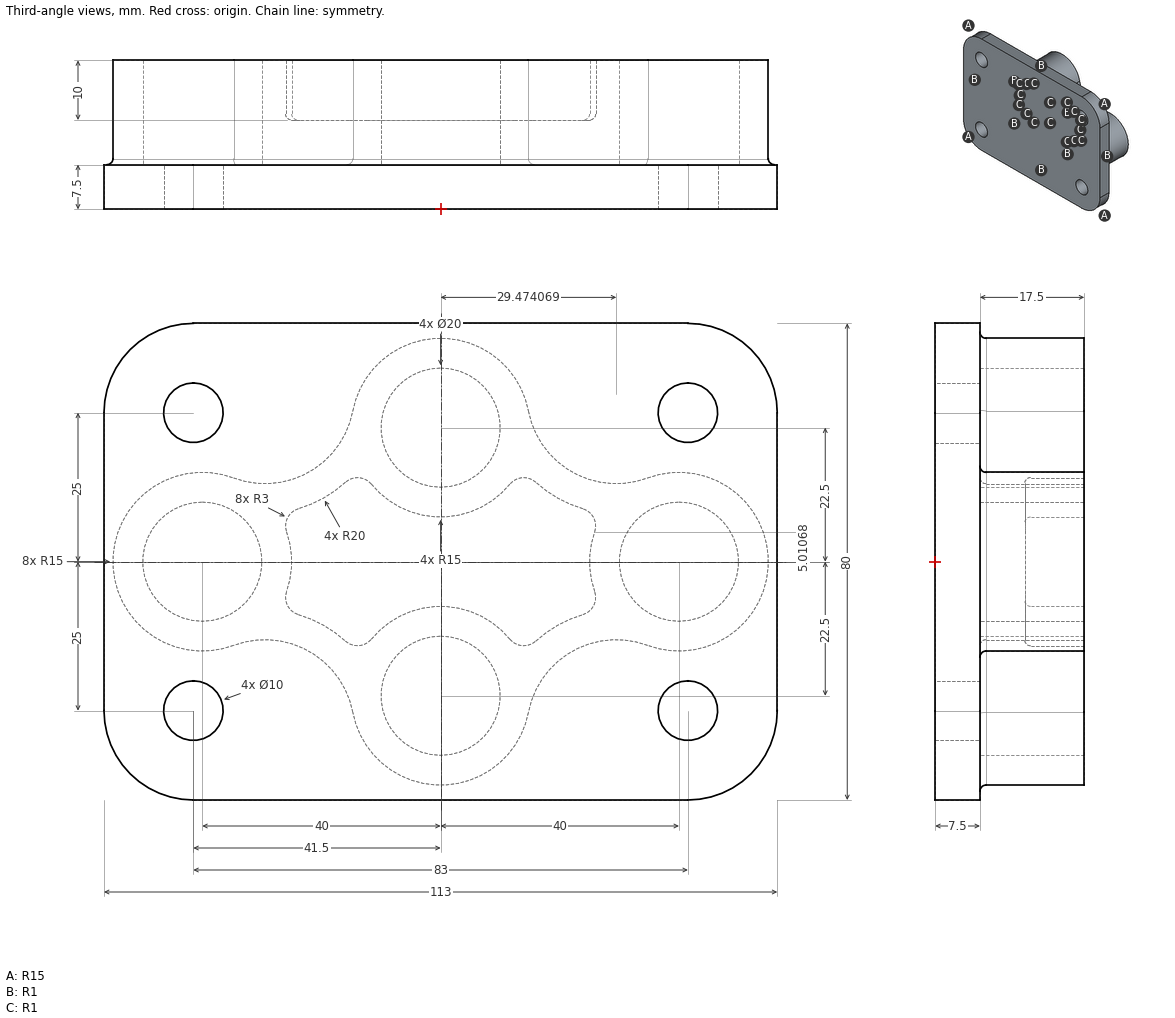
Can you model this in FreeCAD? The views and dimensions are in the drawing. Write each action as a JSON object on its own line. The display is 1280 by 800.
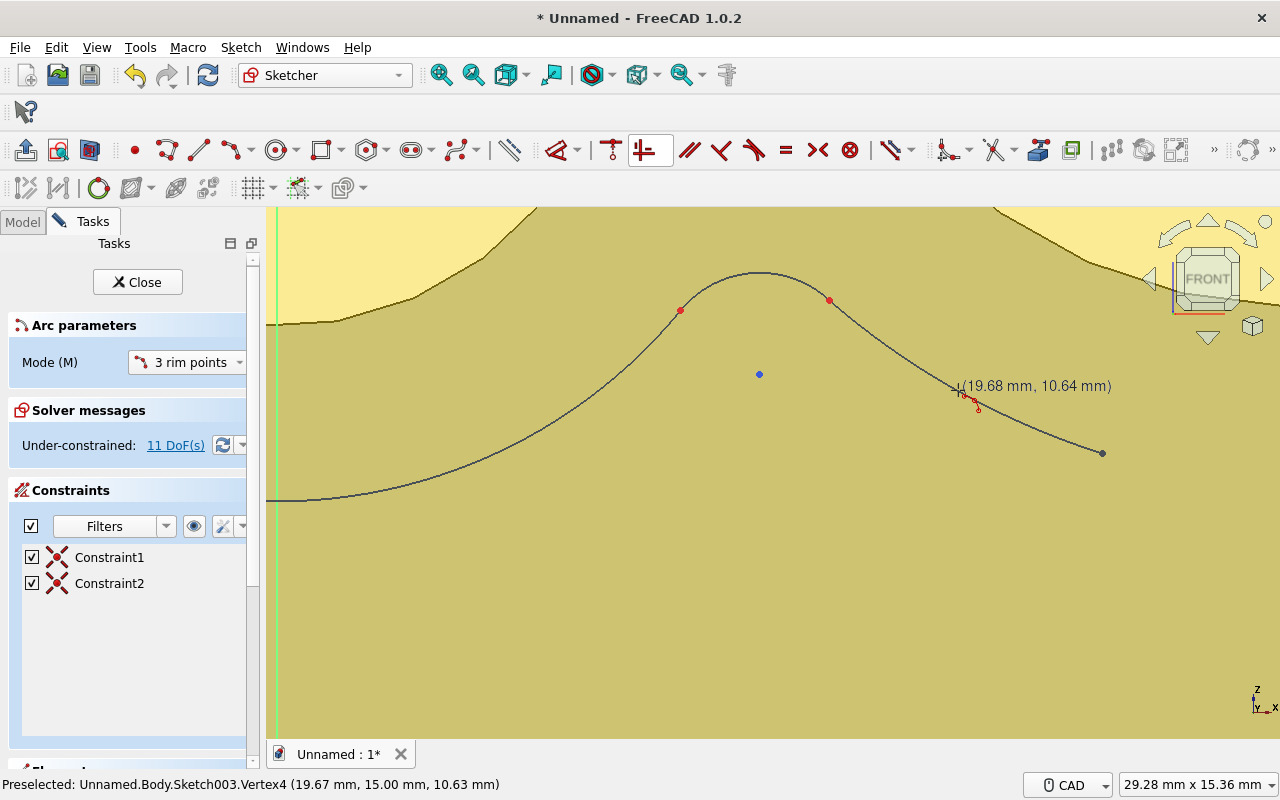
{"action": "left_click", "coordinate": [1102, 453]}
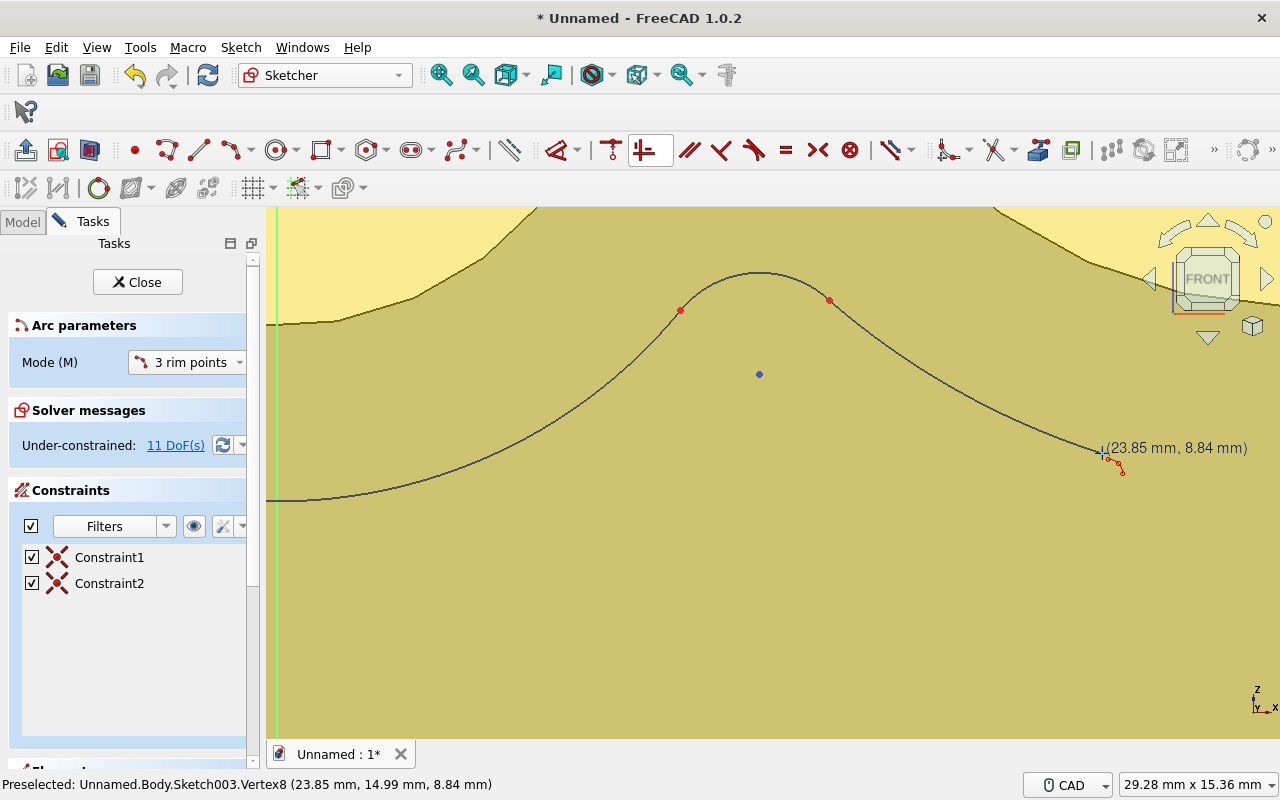
{"action": "scroll", "coordinate": [889, 350], "scroll_direction": "down", "scroll_amount": 6}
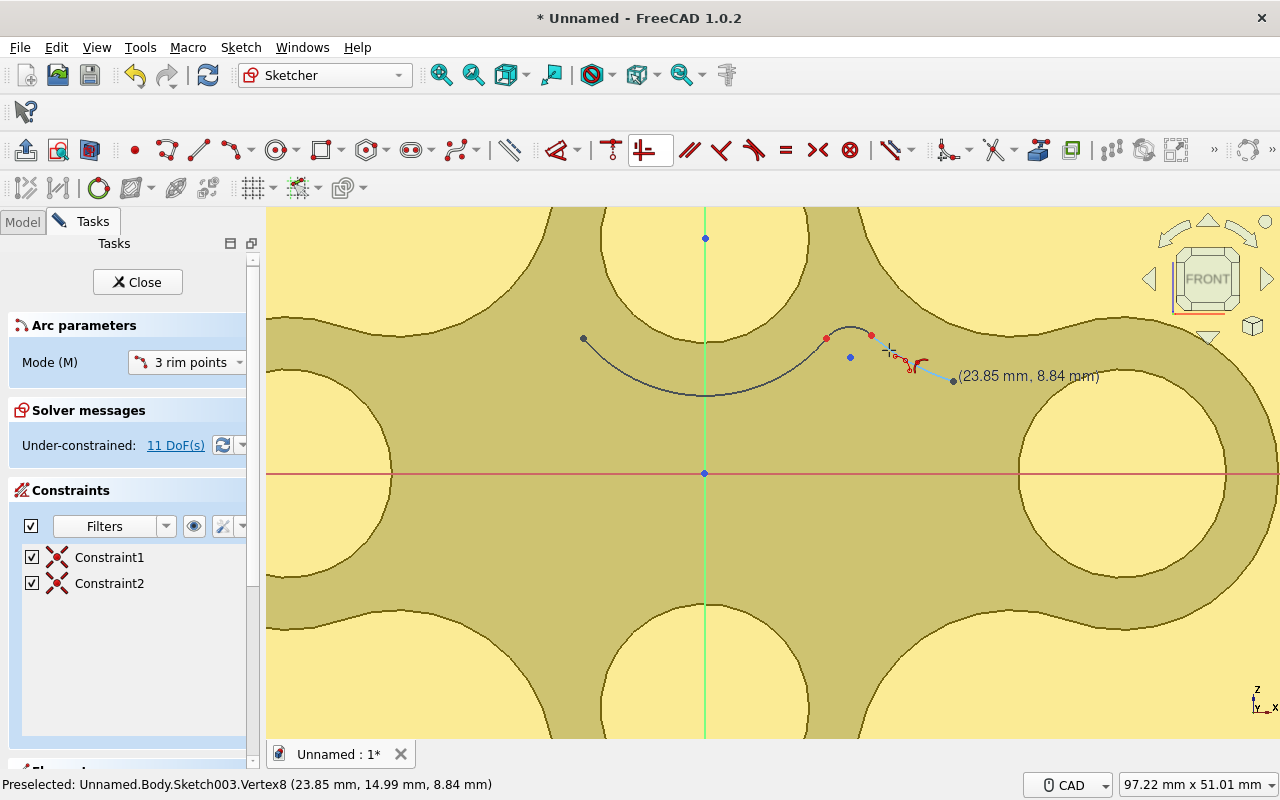
{"action": "left_click", "coordinate": [975, 421]}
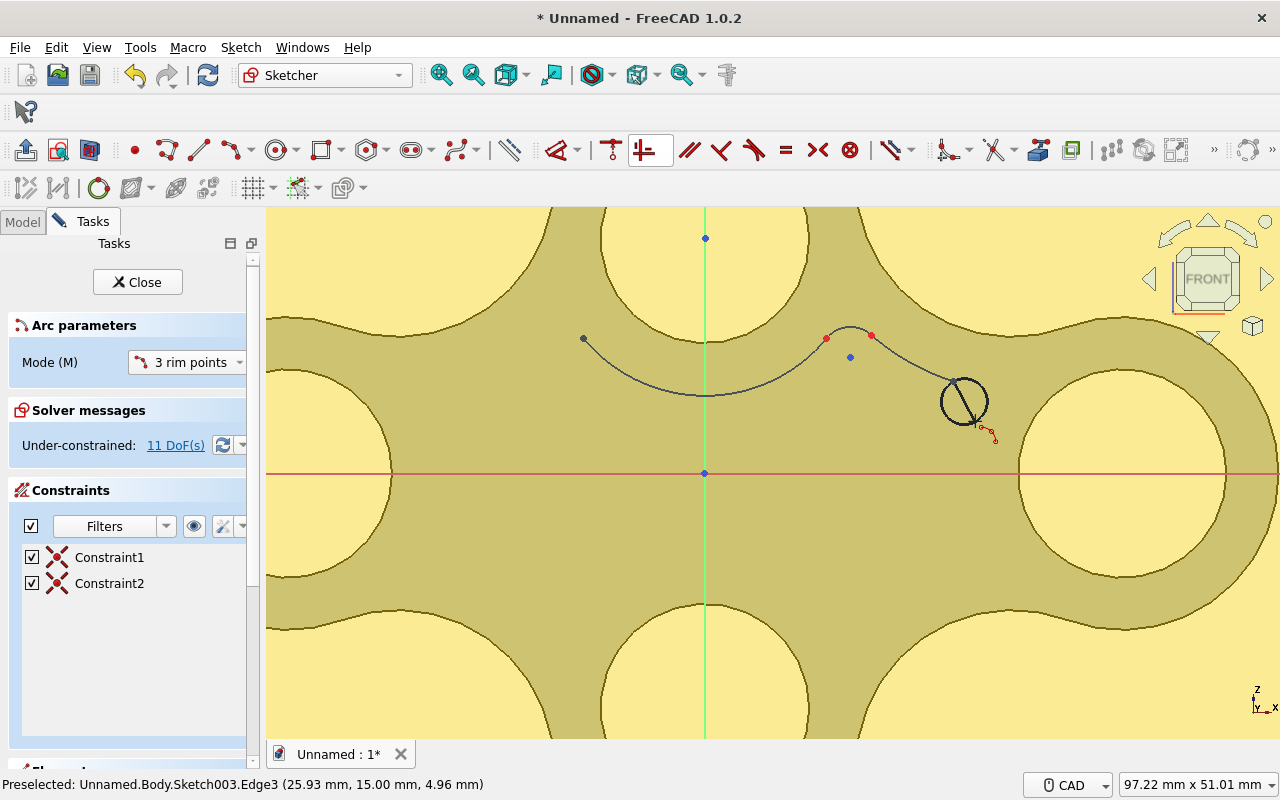
{"action": "scroll", "coordinate": [973, 397], "scroll_direction": "up", "scroll_amount": 3}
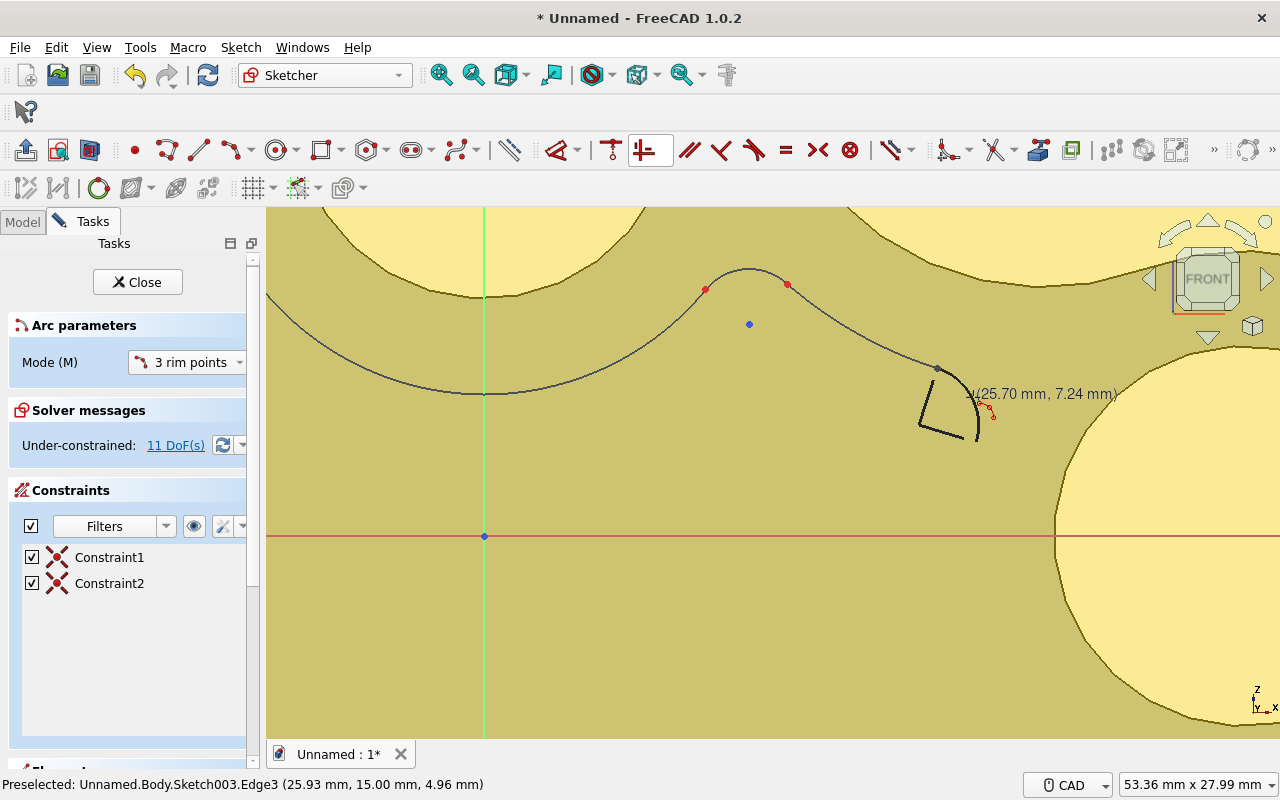
{"action": "left_click", "coordinate": [973, 396]}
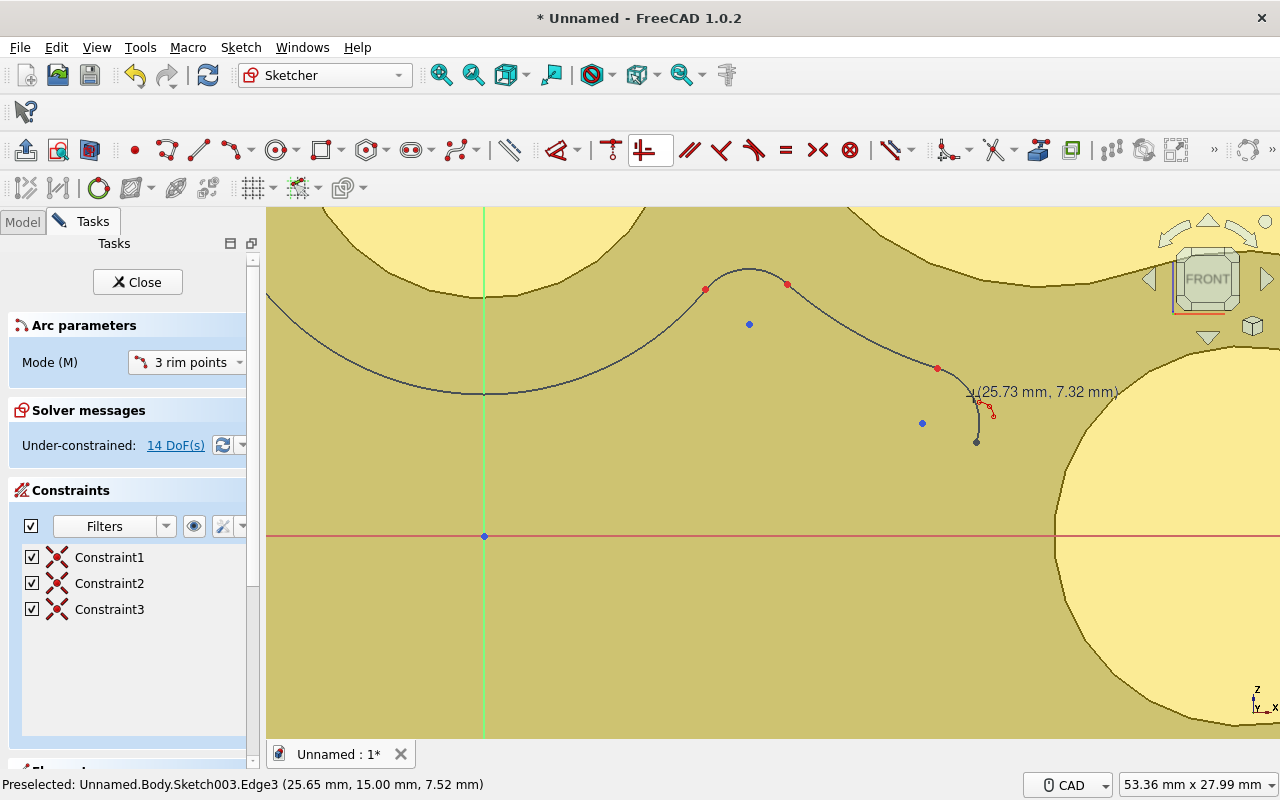
{"action": "left_click", "coordinate": [976, 442]}
{"action": "left_click", "coordinate": [976, 631]}
{"action": "left_click", "coordinate": [960, 517]}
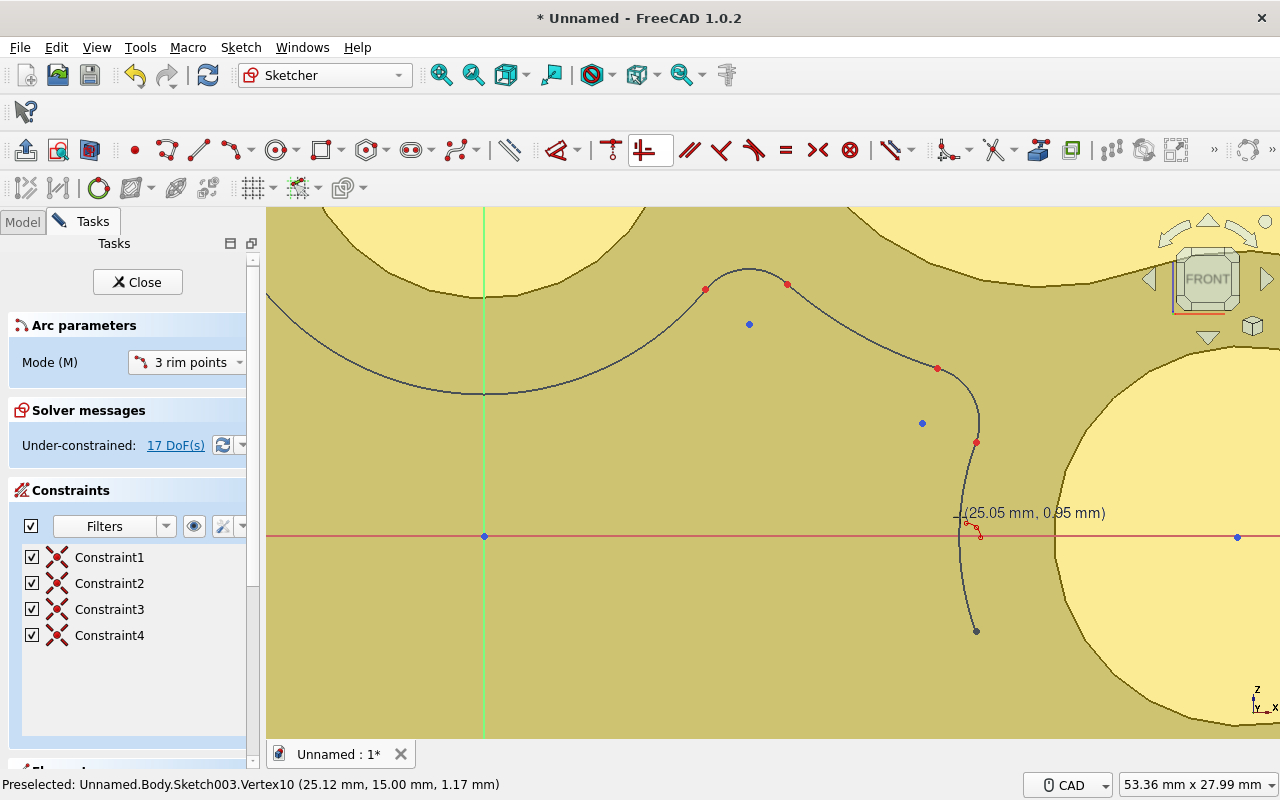
{"action": "left_click", "coordinate": [976, 632]}
{"action": "left_click", "coordinate": [938, 705]}
{"action": "left_click", "coordinate": [973, 676]}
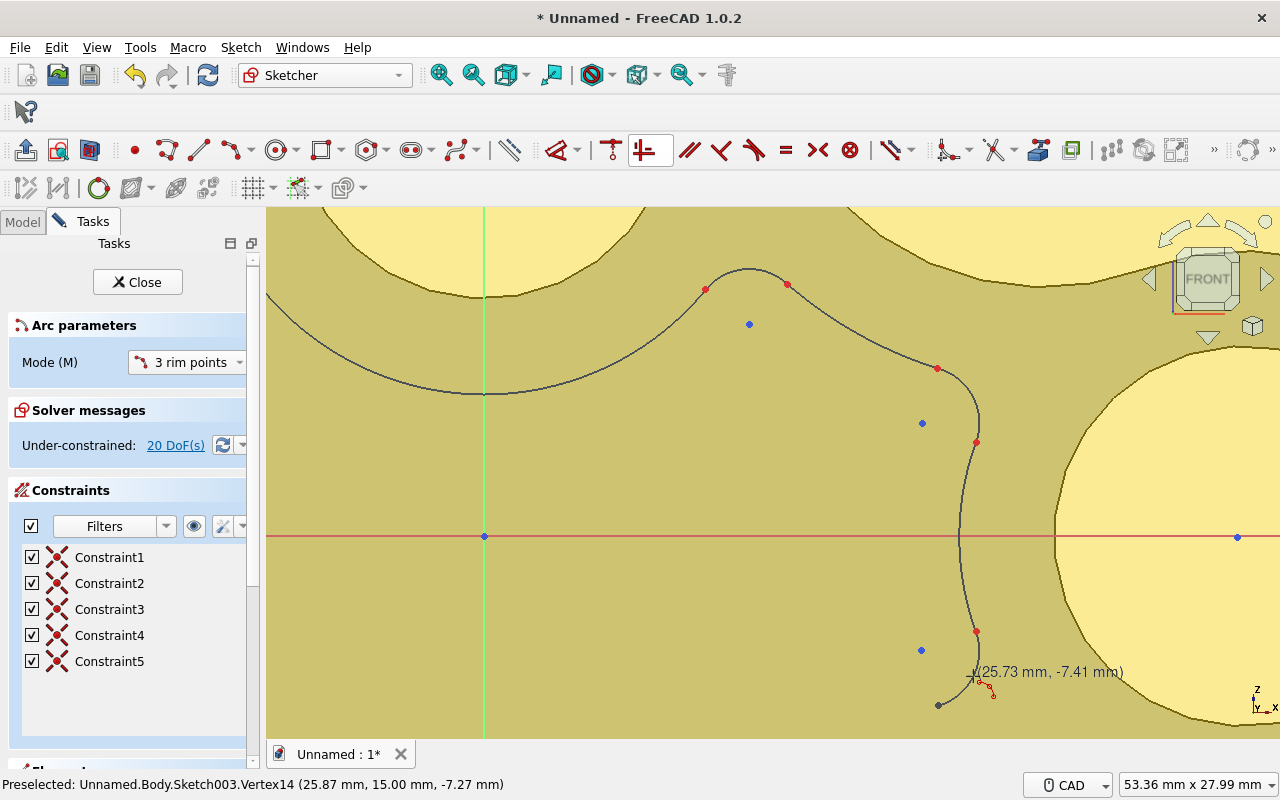
{"action": "left_click", "coordinate": [938, 706]}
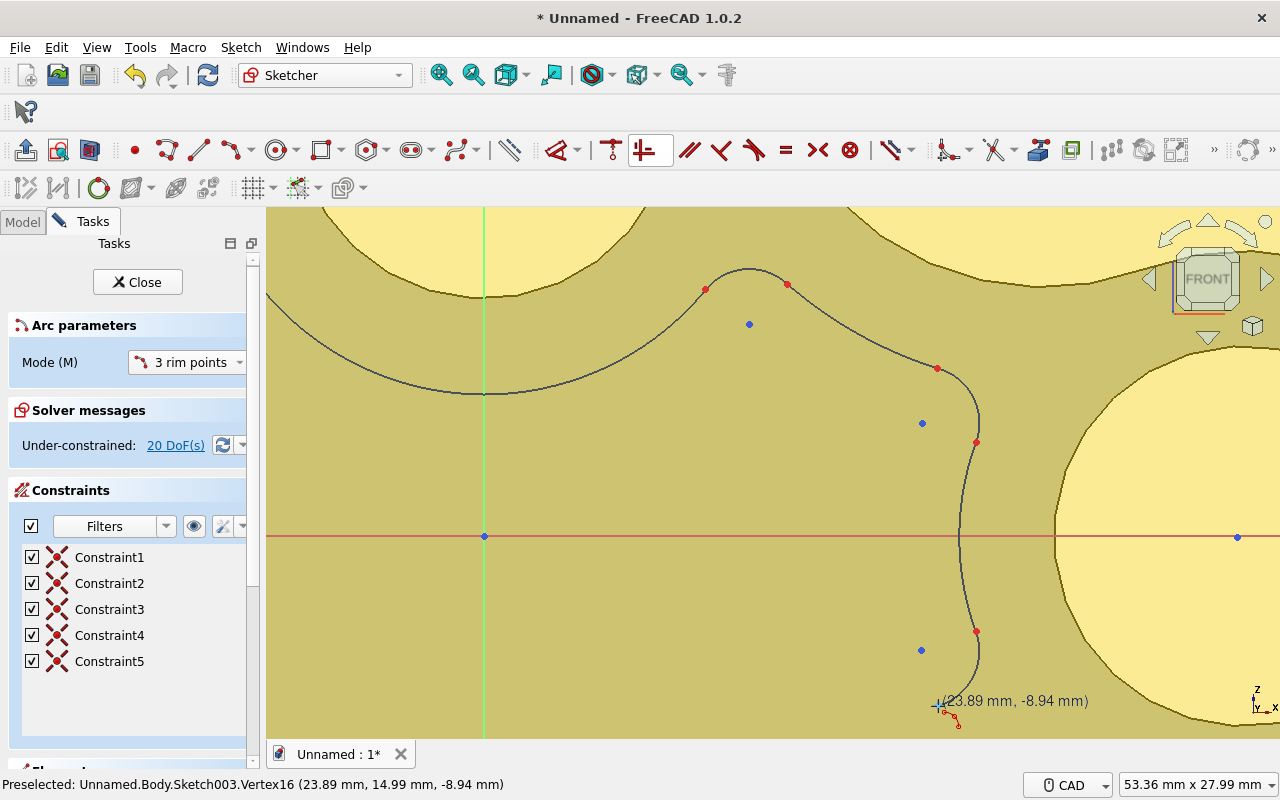
{"action": "scroll", "coordinate": [973, 396], "scroll_direction": "down", "scroll_amount": 3}